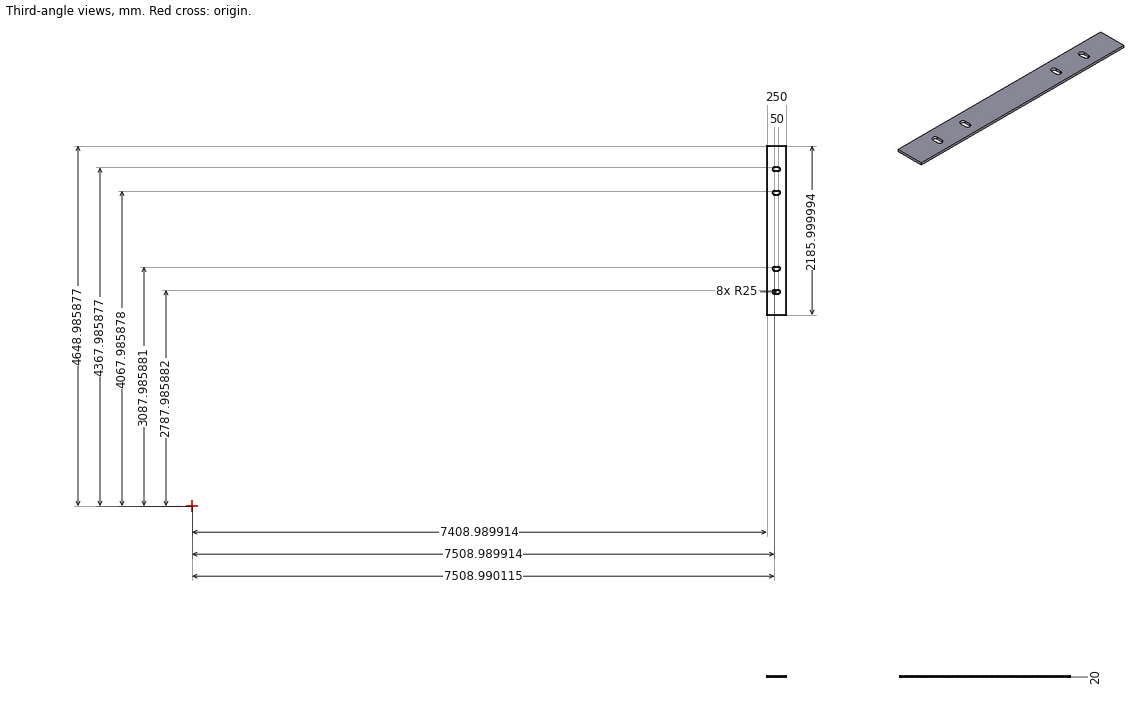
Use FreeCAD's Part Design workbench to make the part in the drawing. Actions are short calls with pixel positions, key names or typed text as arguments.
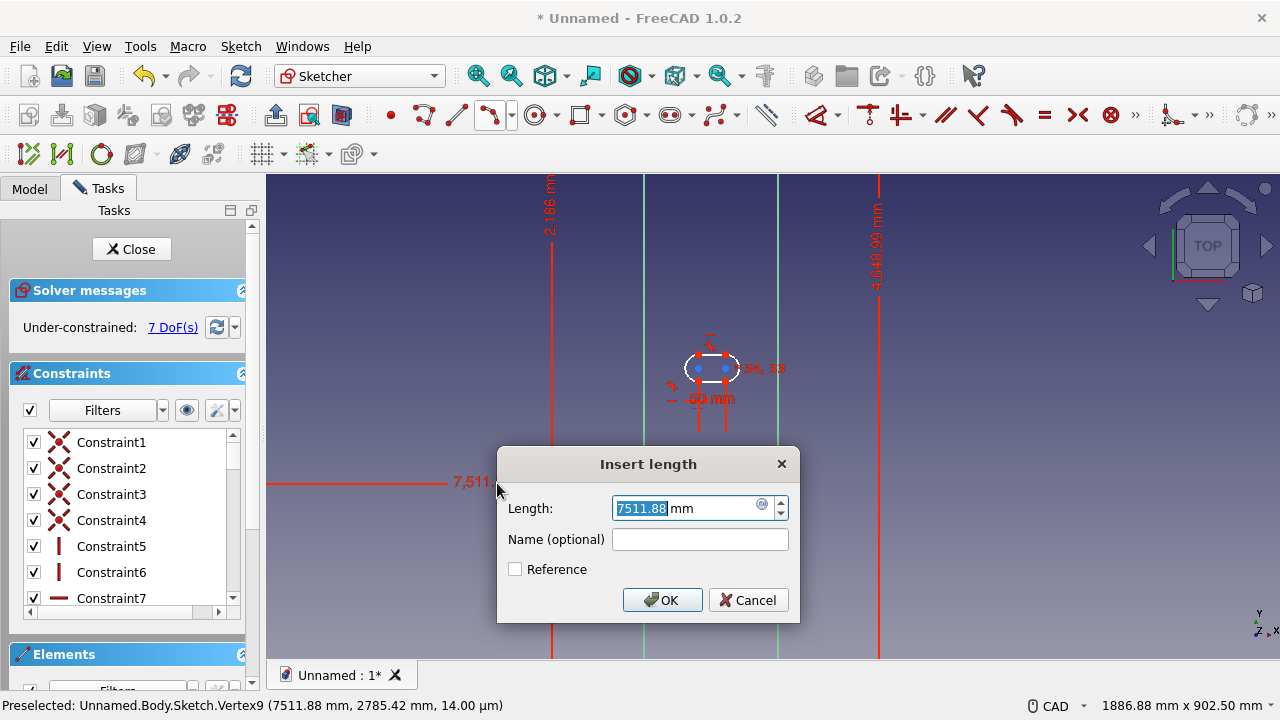
text(7508.989914)
key(Return)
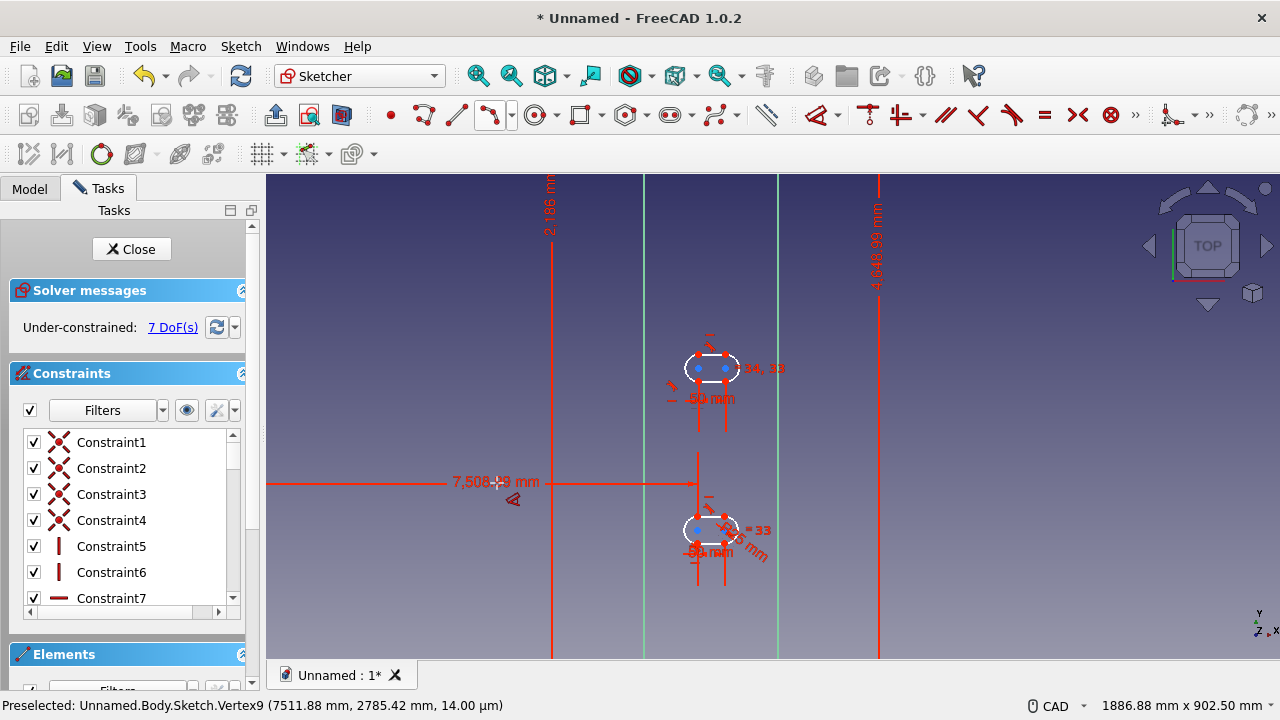
click(698, 517)
click(732, 600)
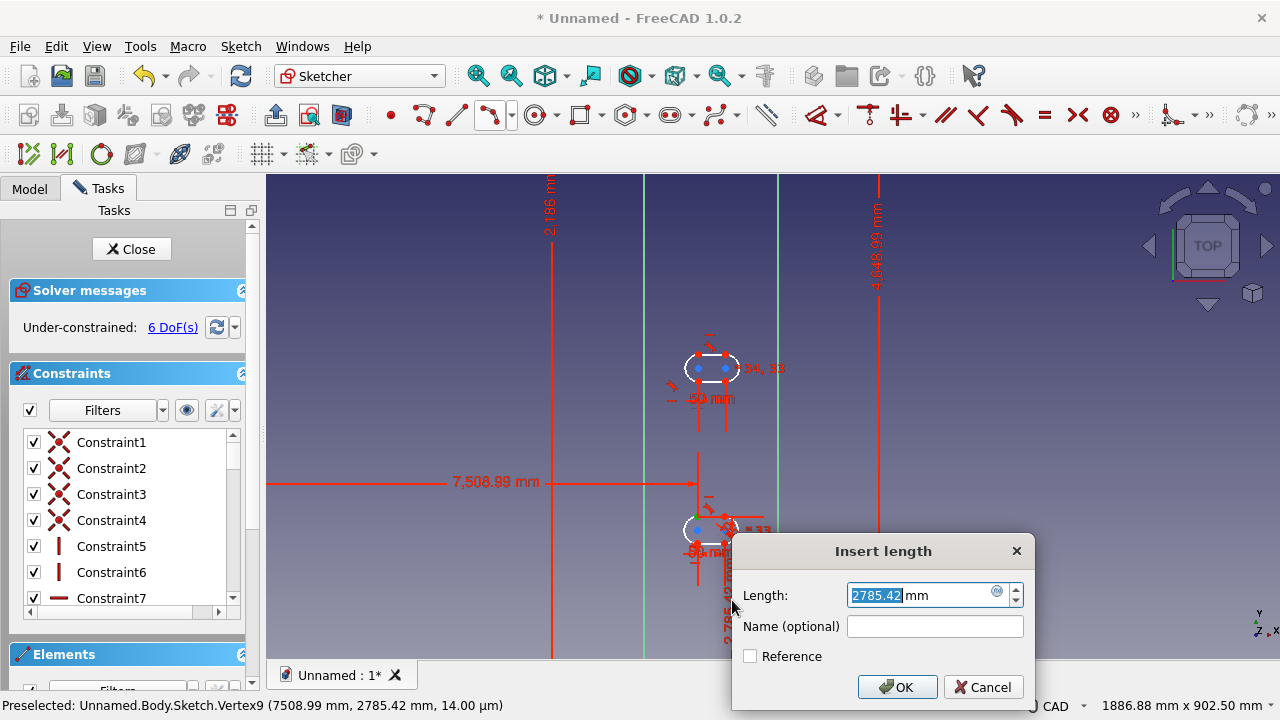
text(2787.985882)
key(Return)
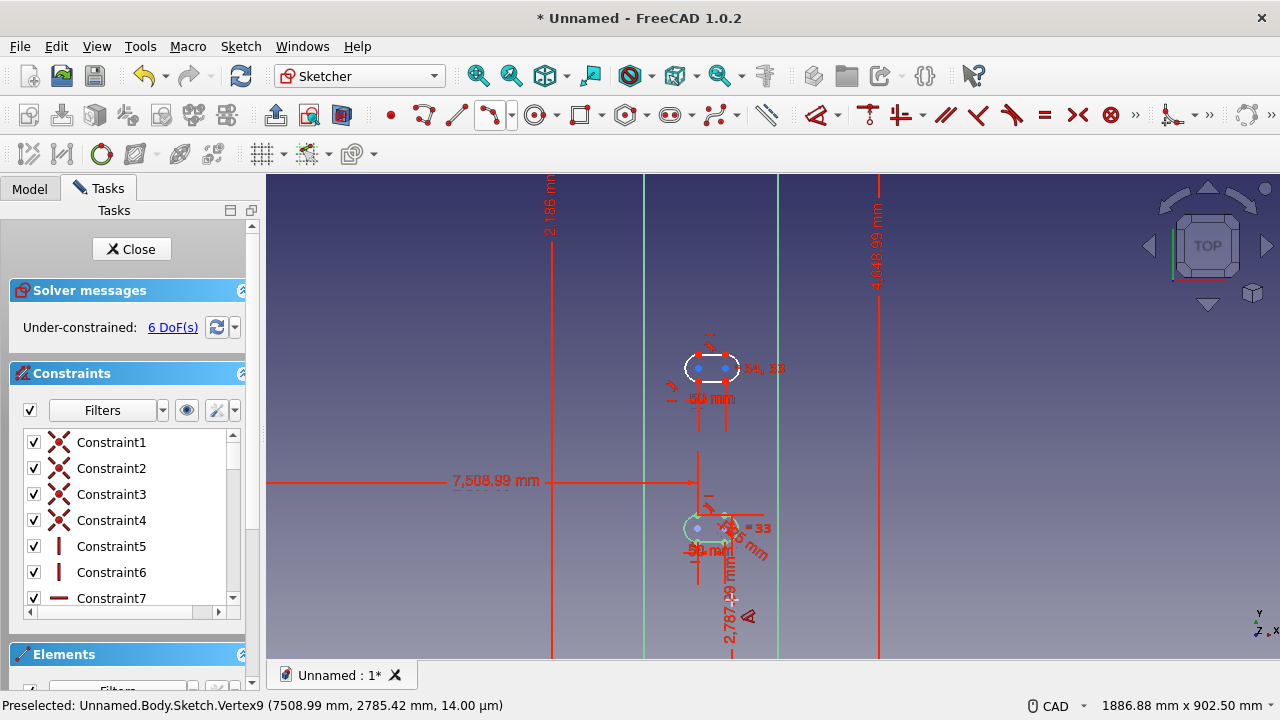
click(699, 355)
click(496, 321)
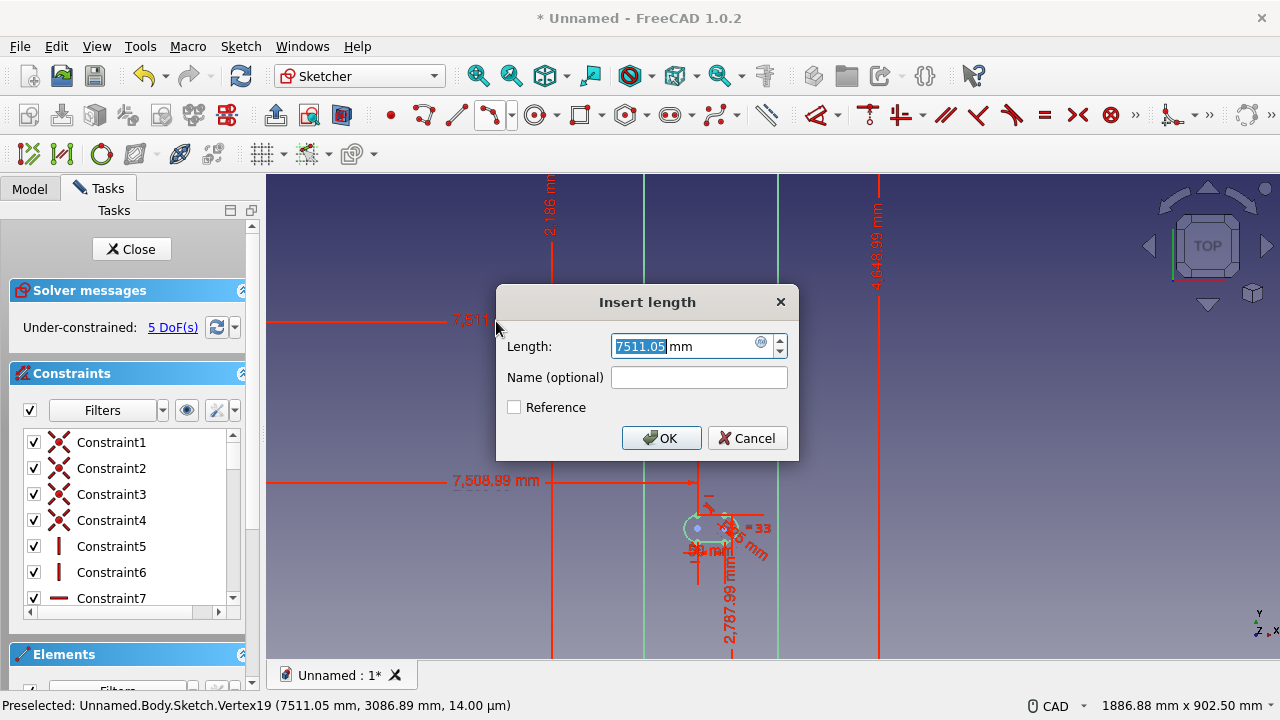
text(7508.990115)
key(Return)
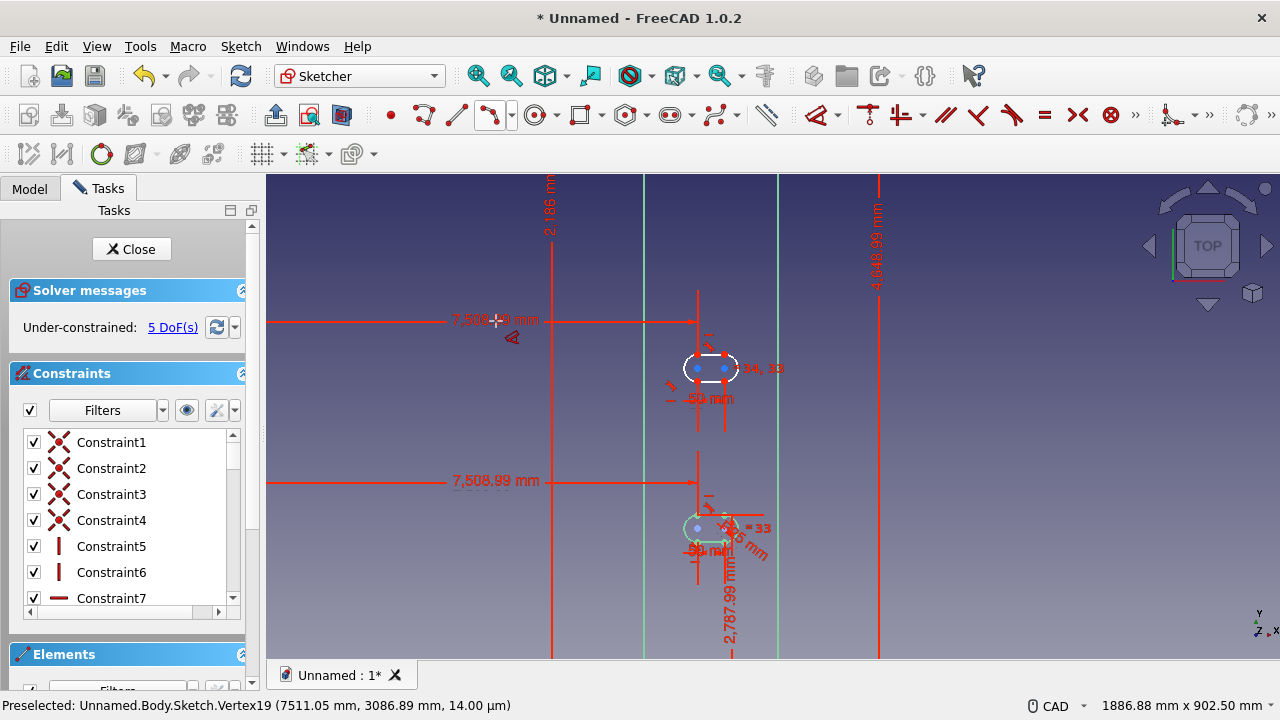
click(698, 355)
click(732, 493)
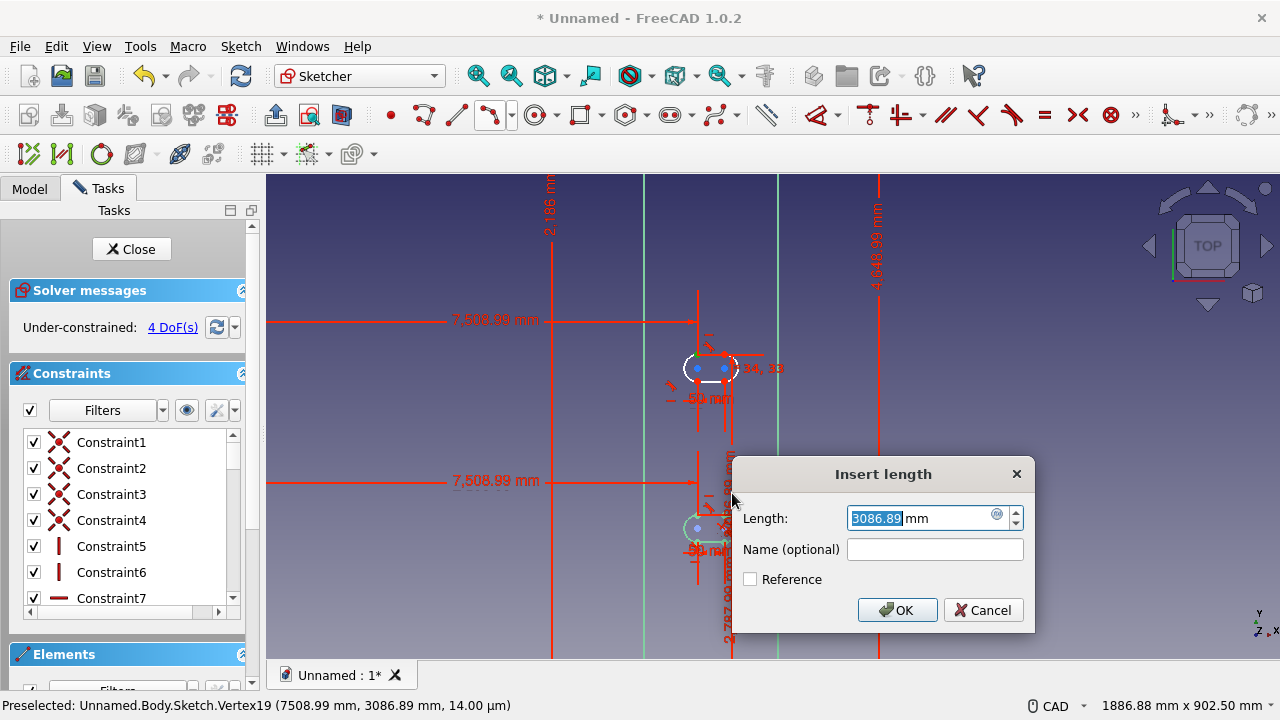
text(3087.985881)
key(Return)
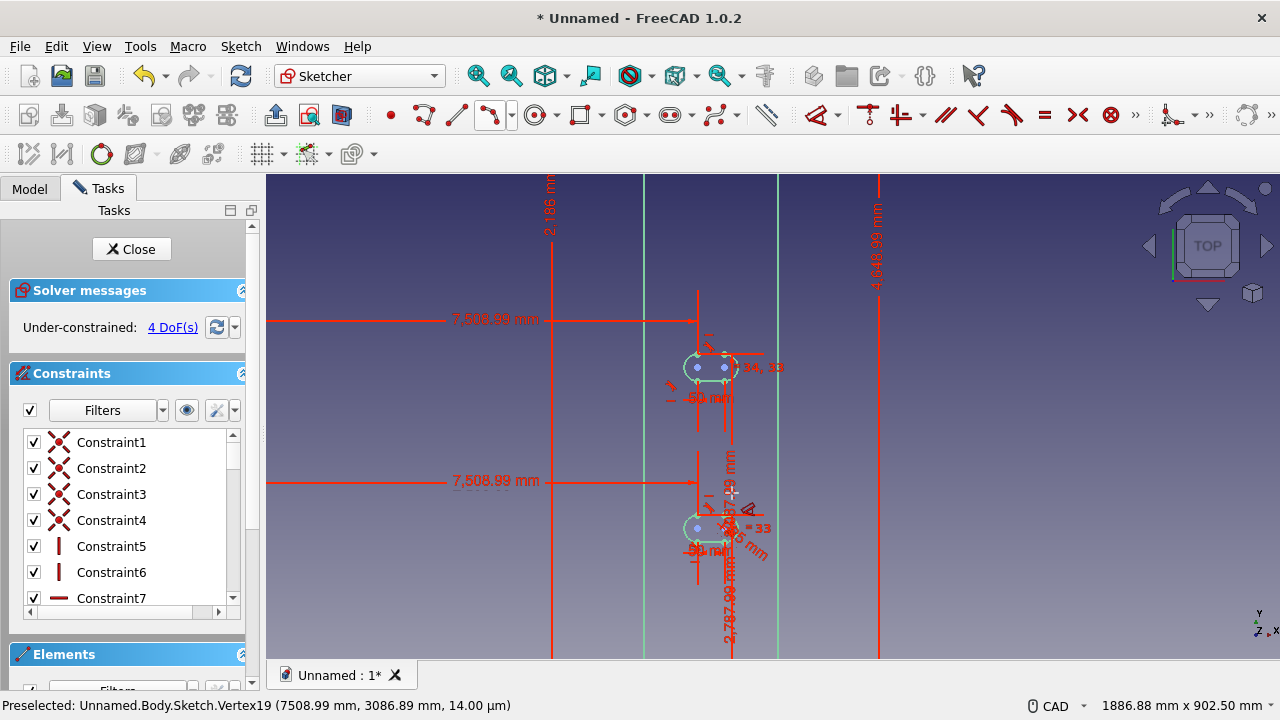
scroll(702, 519, down, 7)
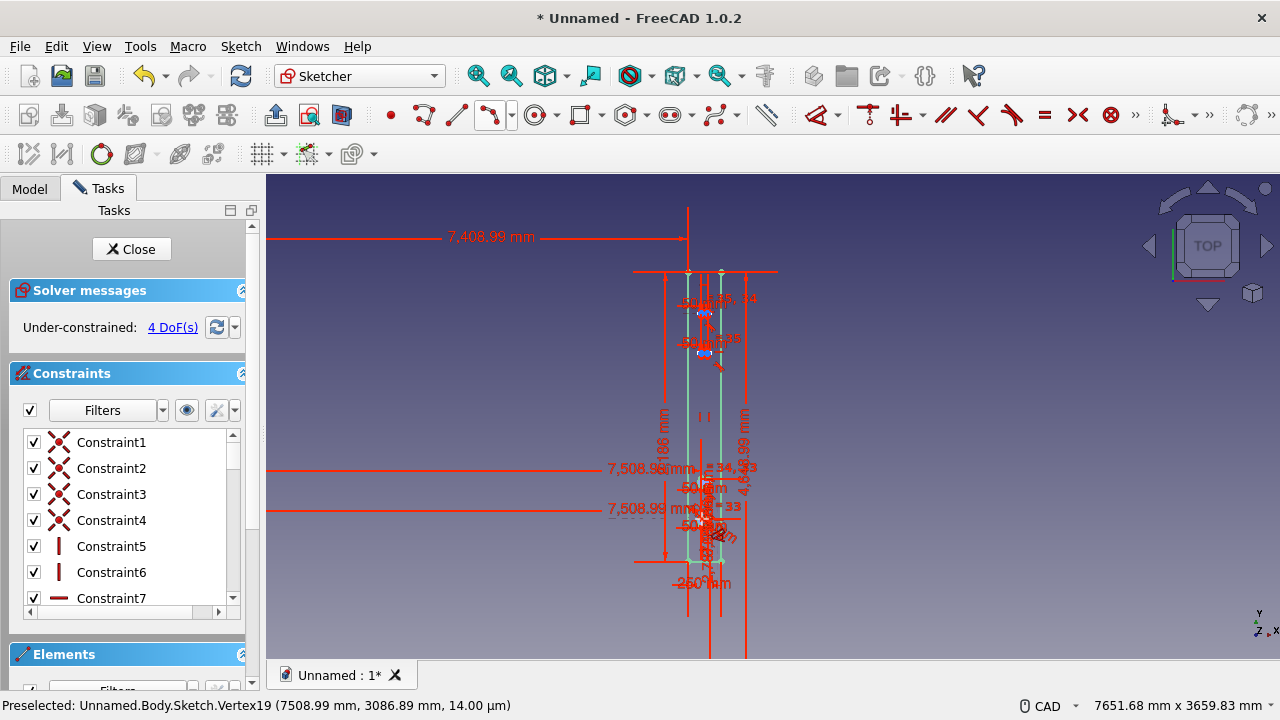
scroll(701, 310, up, 7)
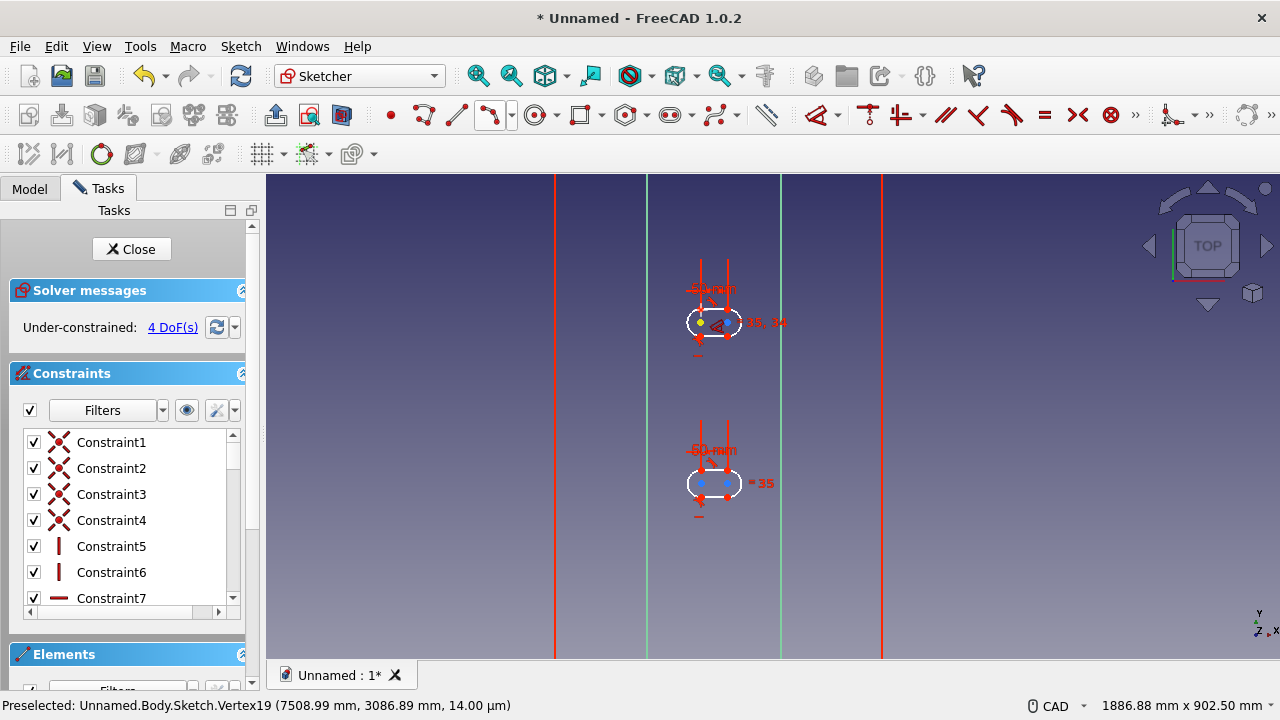
click(701, 309)
click(497, 275)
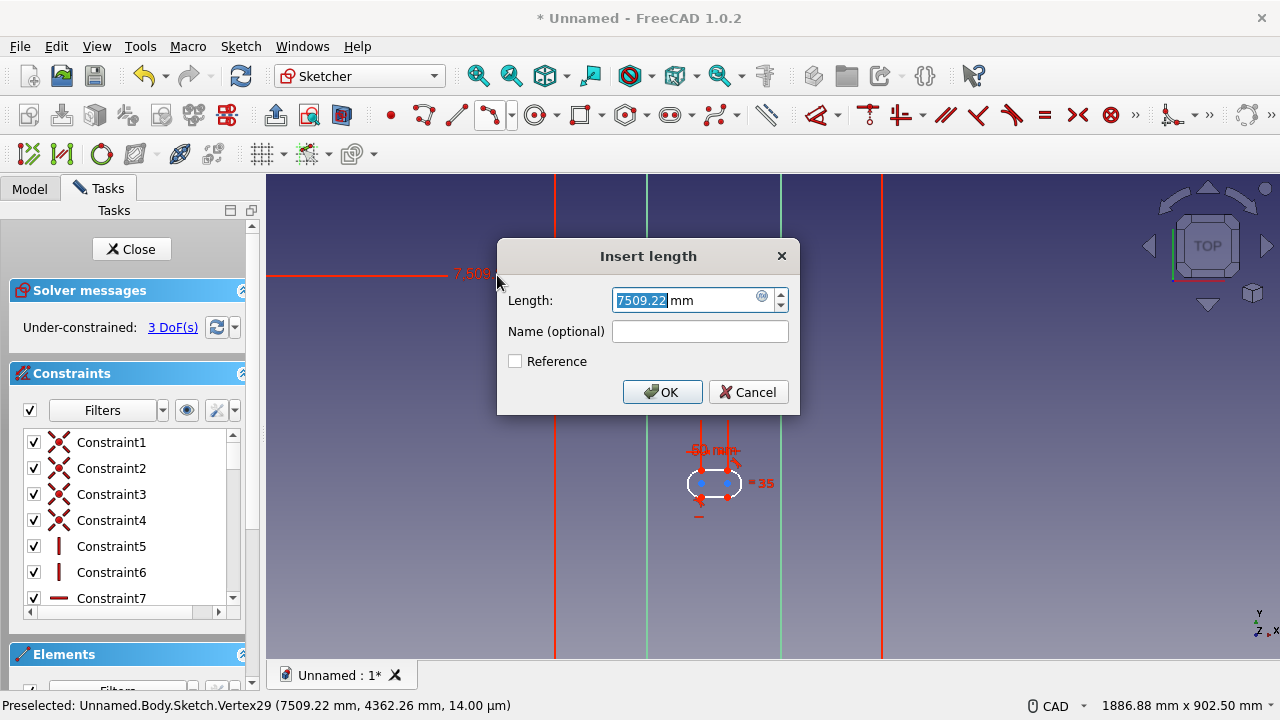
text(7508.989914)
key(Return)